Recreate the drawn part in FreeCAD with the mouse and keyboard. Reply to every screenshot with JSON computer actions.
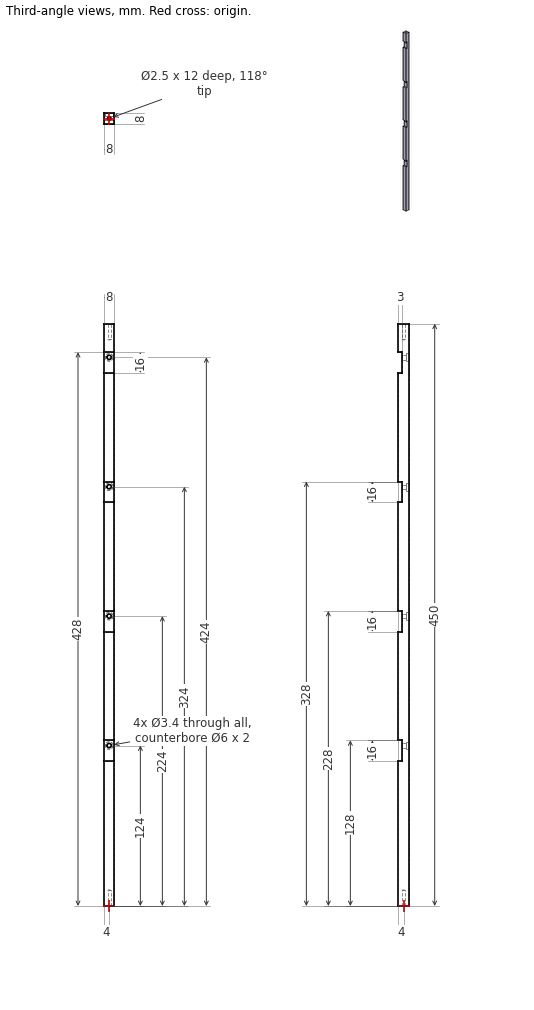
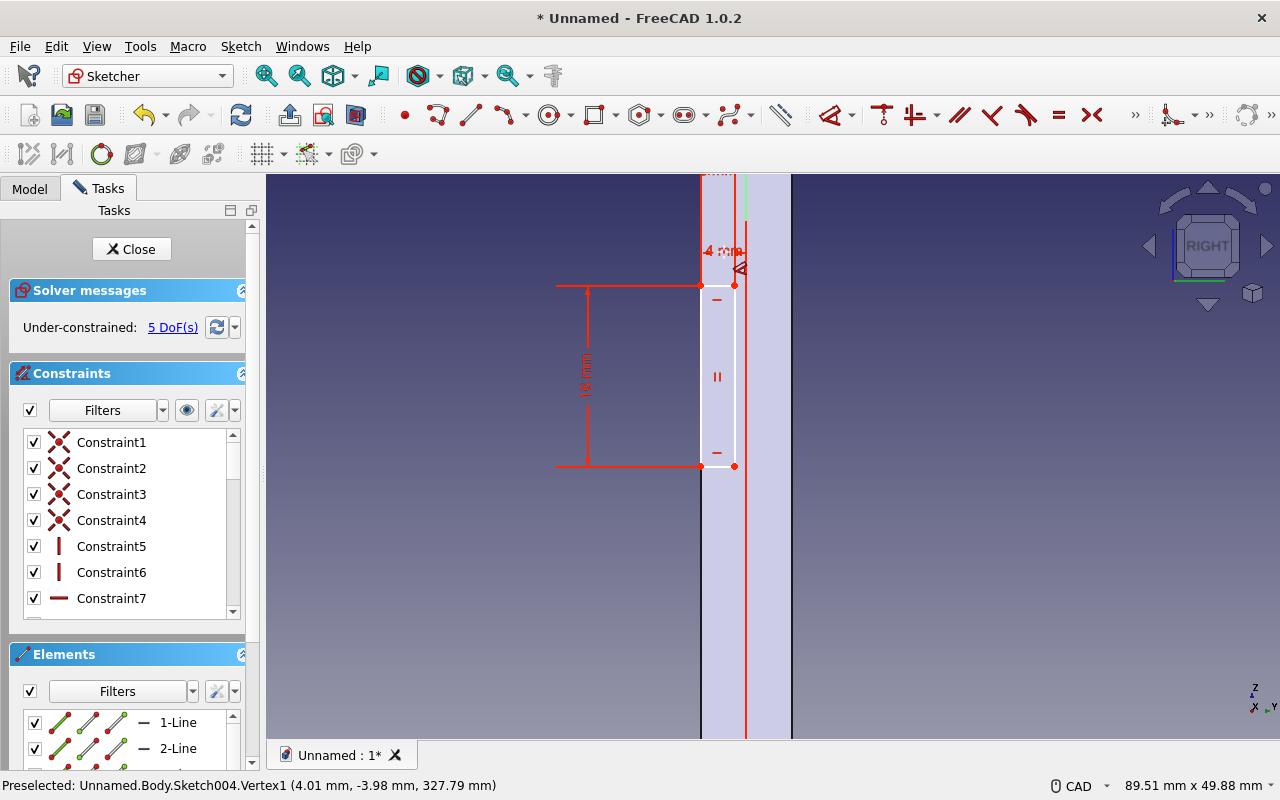
{"action": "scroll", "coordinate": [703, 288], "scroll_direction": "down", "scroll_amount": 12}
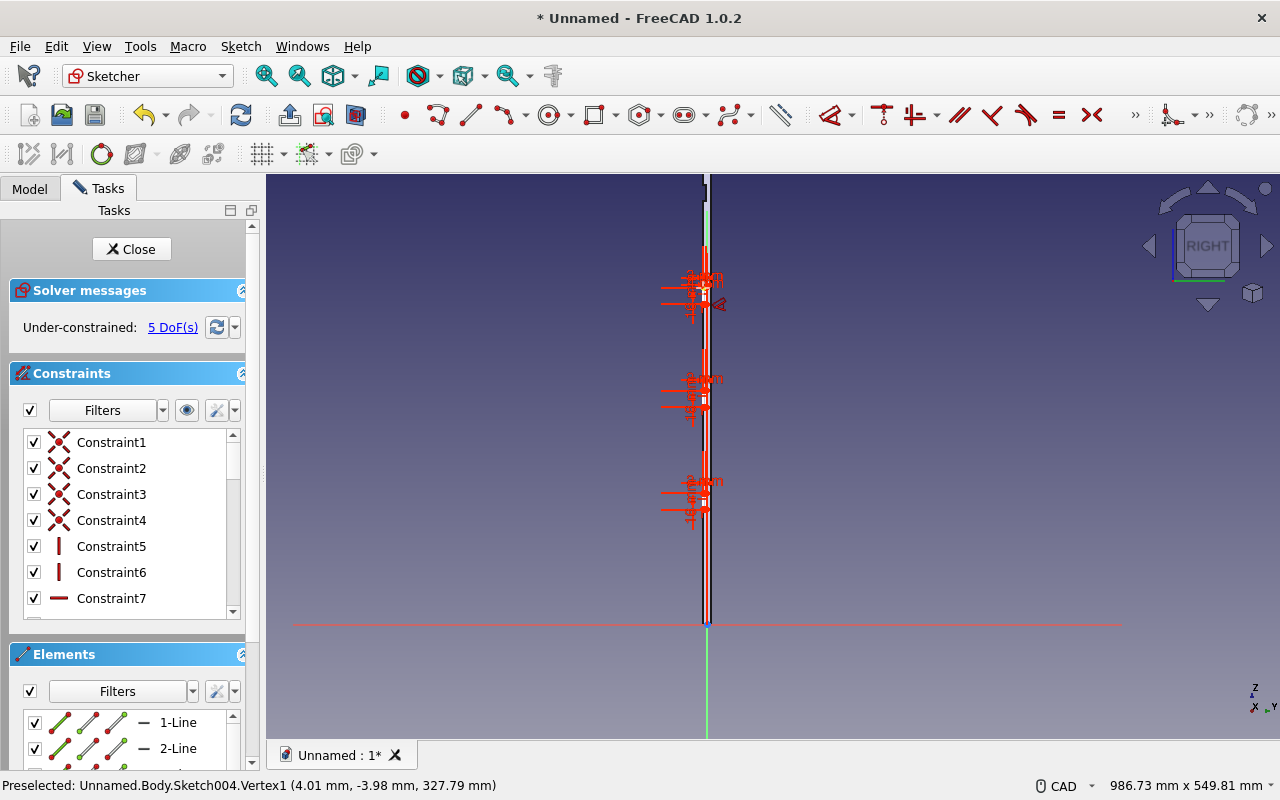
{"action": "scroll", "coordinate": [703, 391], "scroll_direction": "up", "scroll_amount": 12}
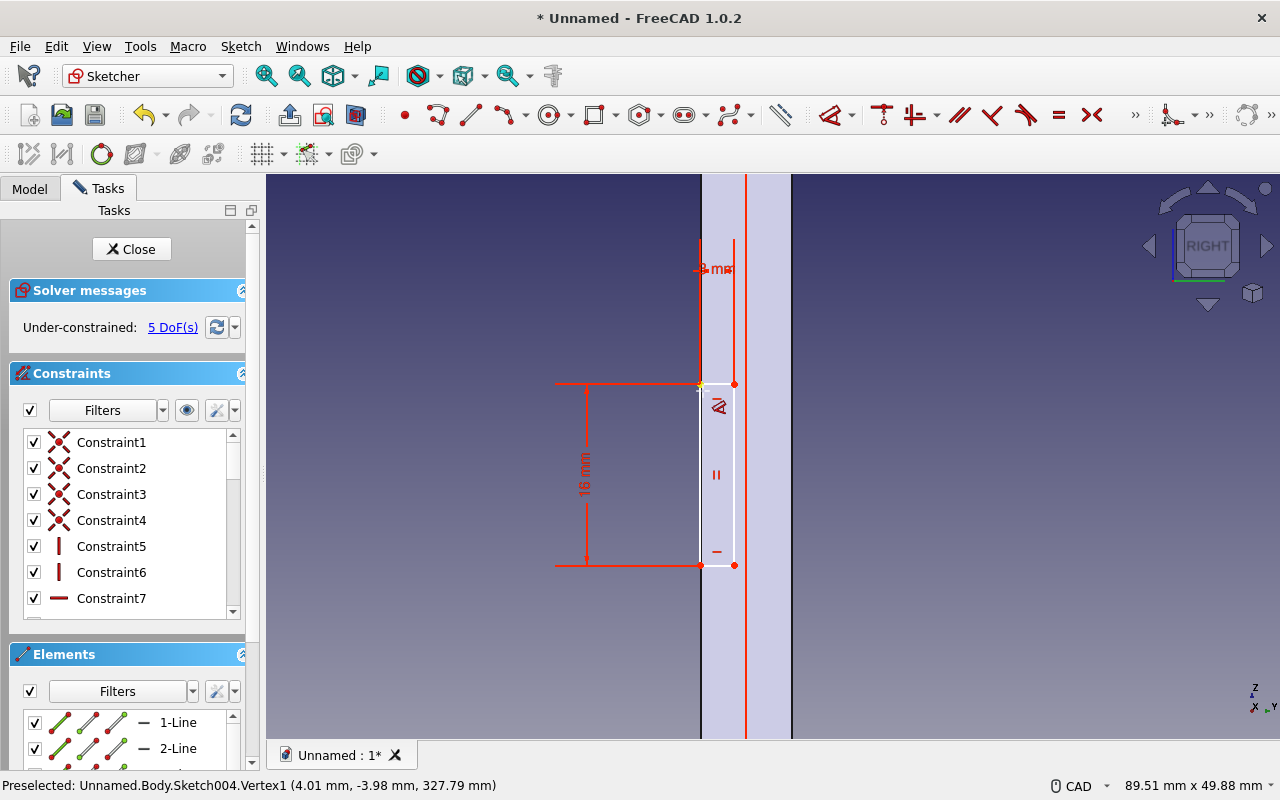
{"action": "left_click", "coordinate": [700, 384]}
{"action": "left_click", "coordinate": [723, 350]}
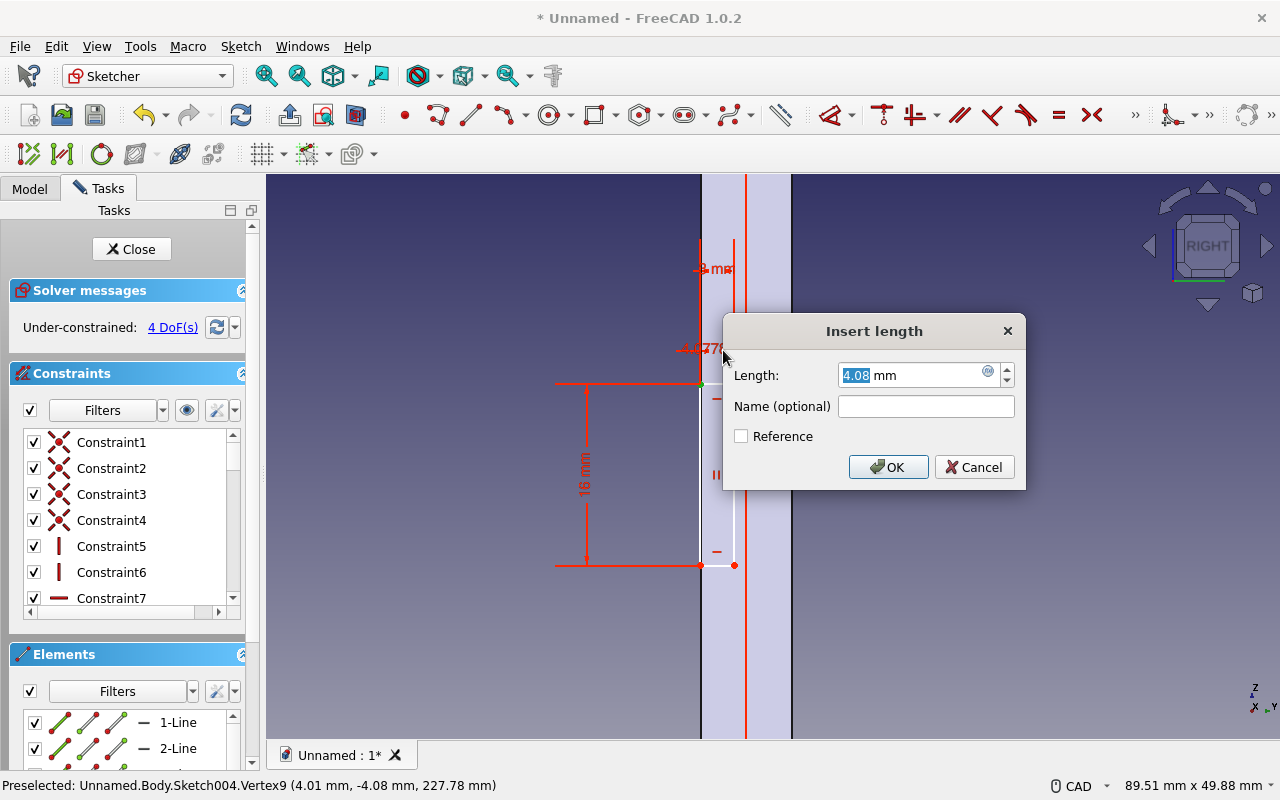
{"action": "type", "text": "4"}
{"action": "key", "text": "Return"}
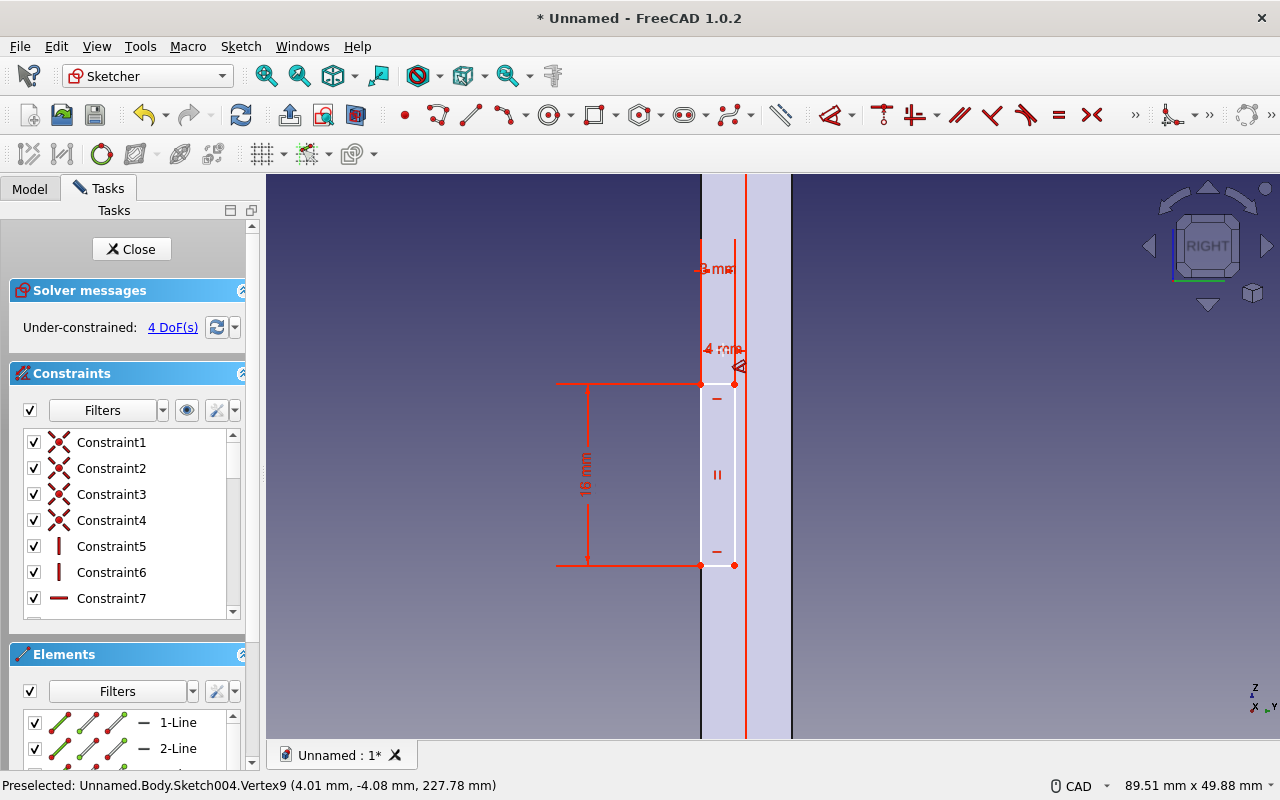
{"action": "scroll", "coordinate": [703, 392], "scroll_direction": "down", "scroll_amount": 12}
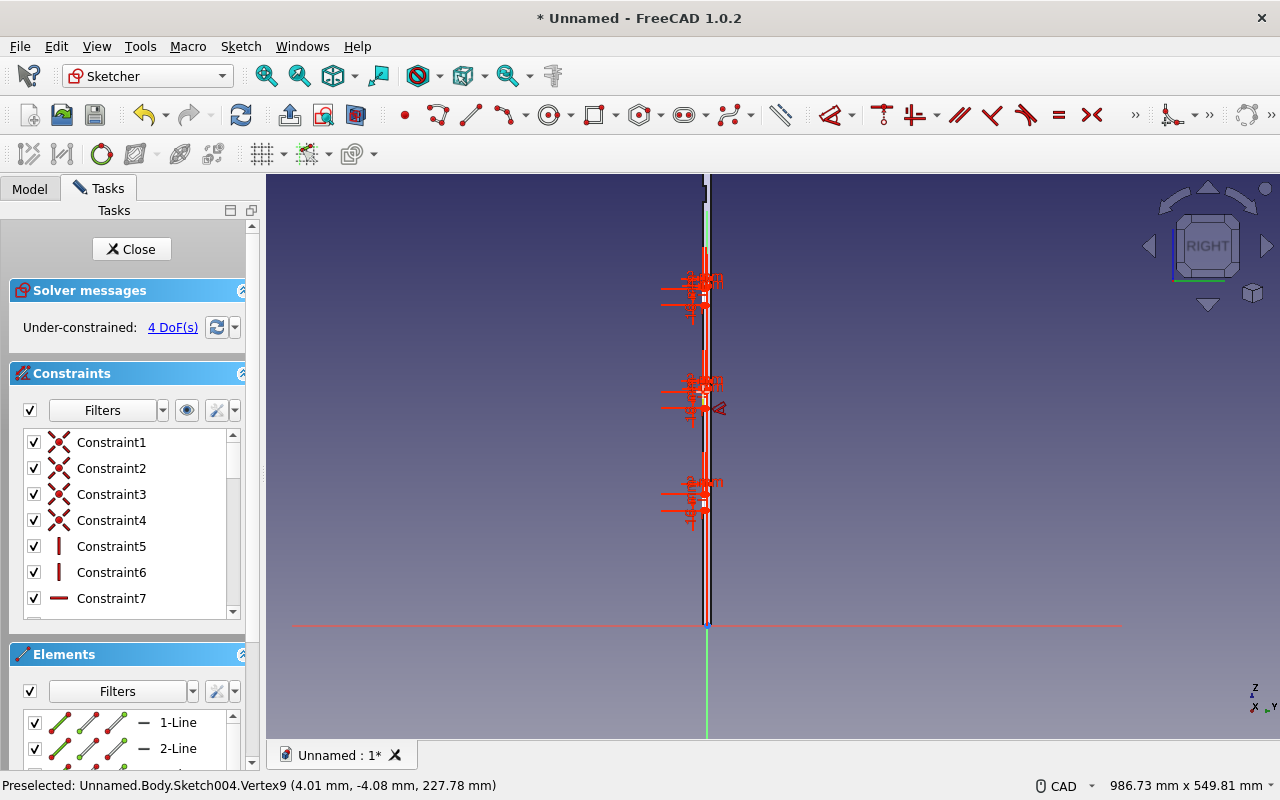
{"action": "scroll", "coordinate": [703, 494], "scroll_direction": "up", "scroll_amount": 12}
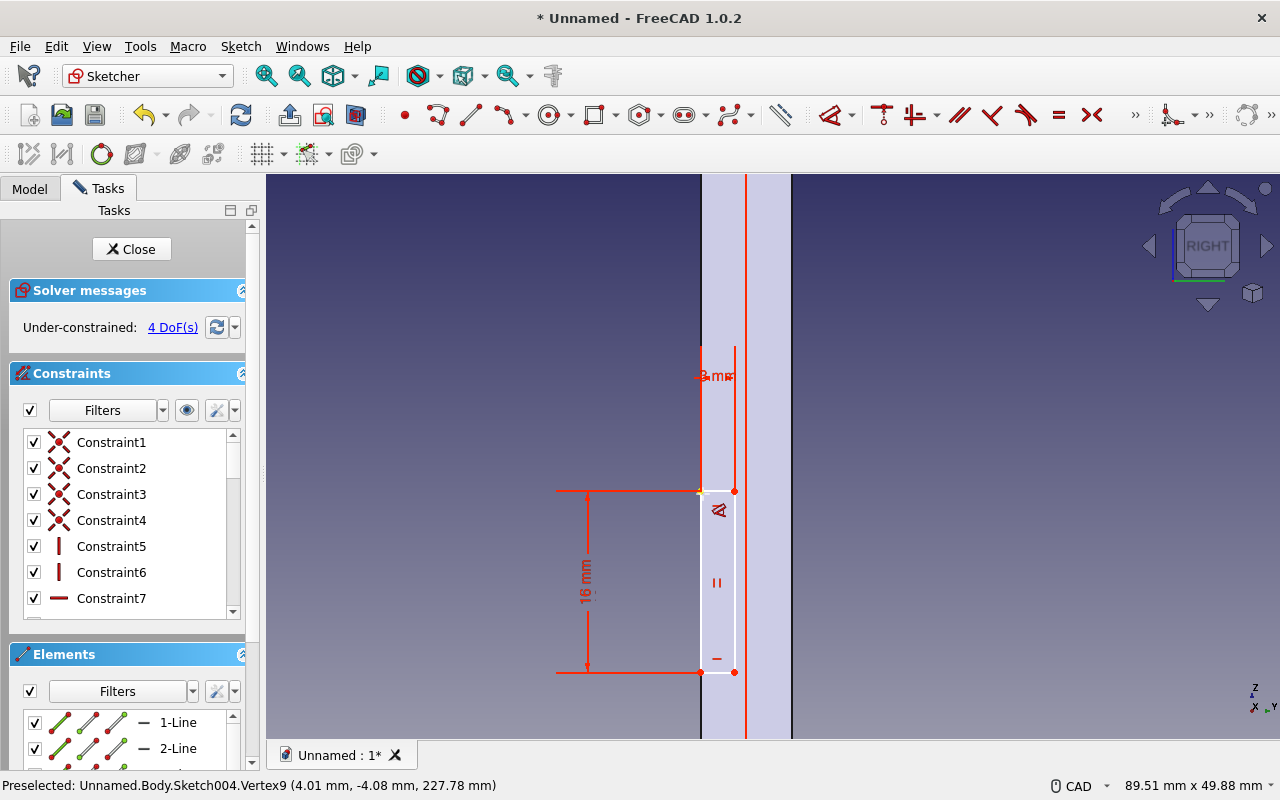
{"action": "left_click", "coordinate": [701, 491]}
{"action": "left_click", "coordinate": [724, 457]}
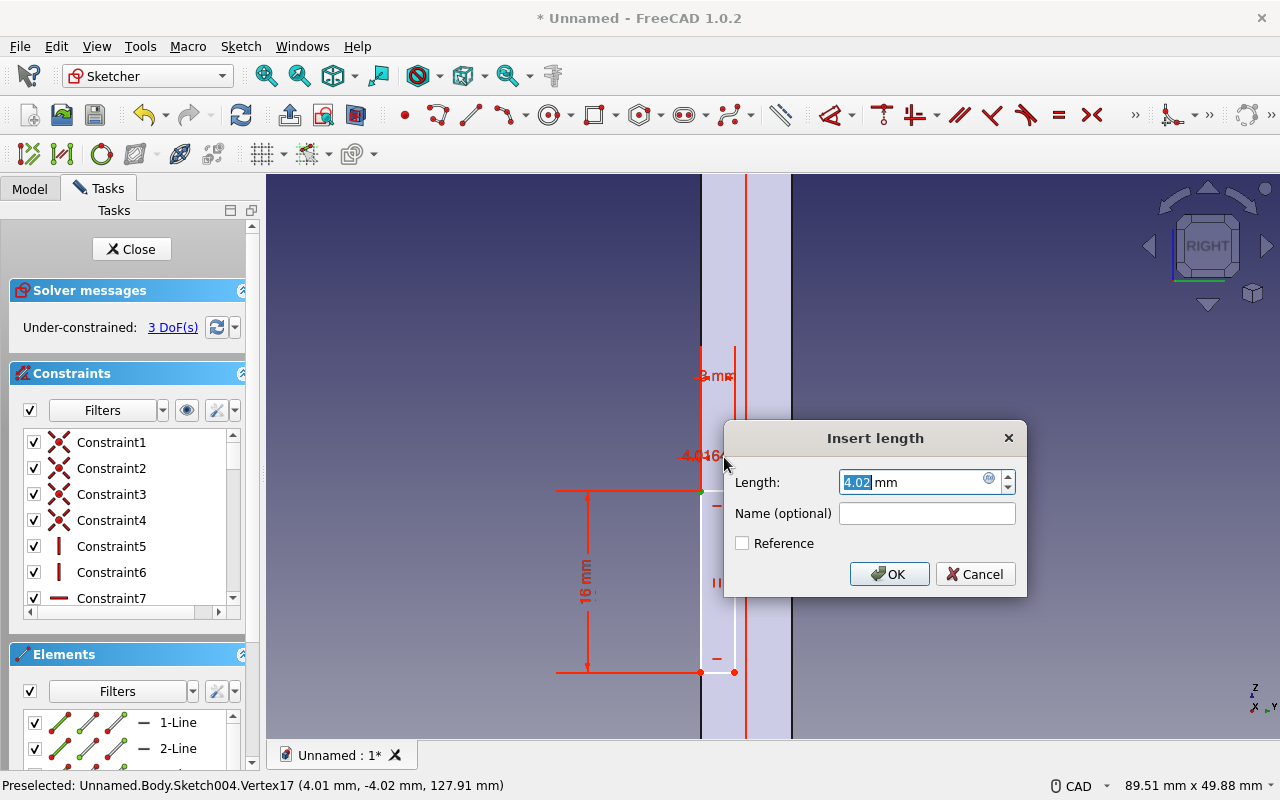
{"action": "type", "text": "4"}
{"action": "key", "text": "Return"}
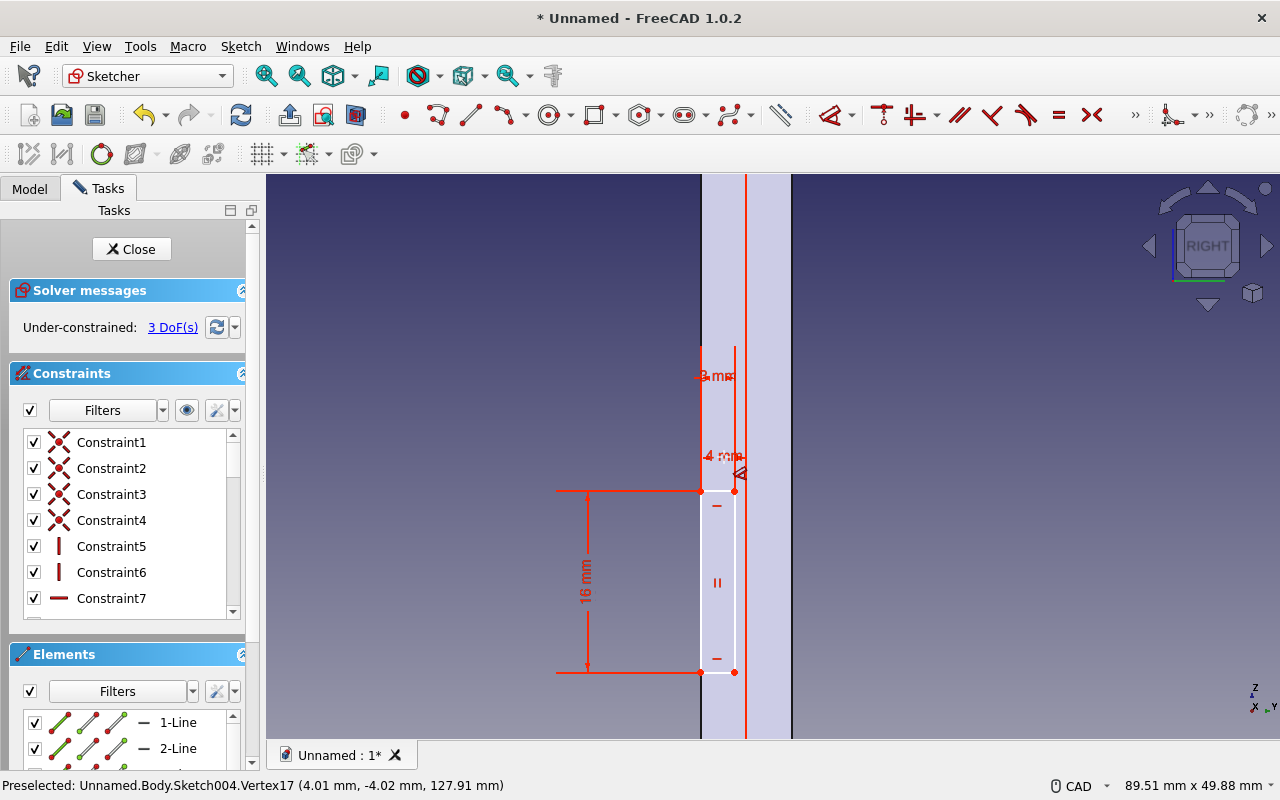
{"action": "scroll", "coordinate": [703, 494], "scroll_direction": "down", "scroll_amount": 12}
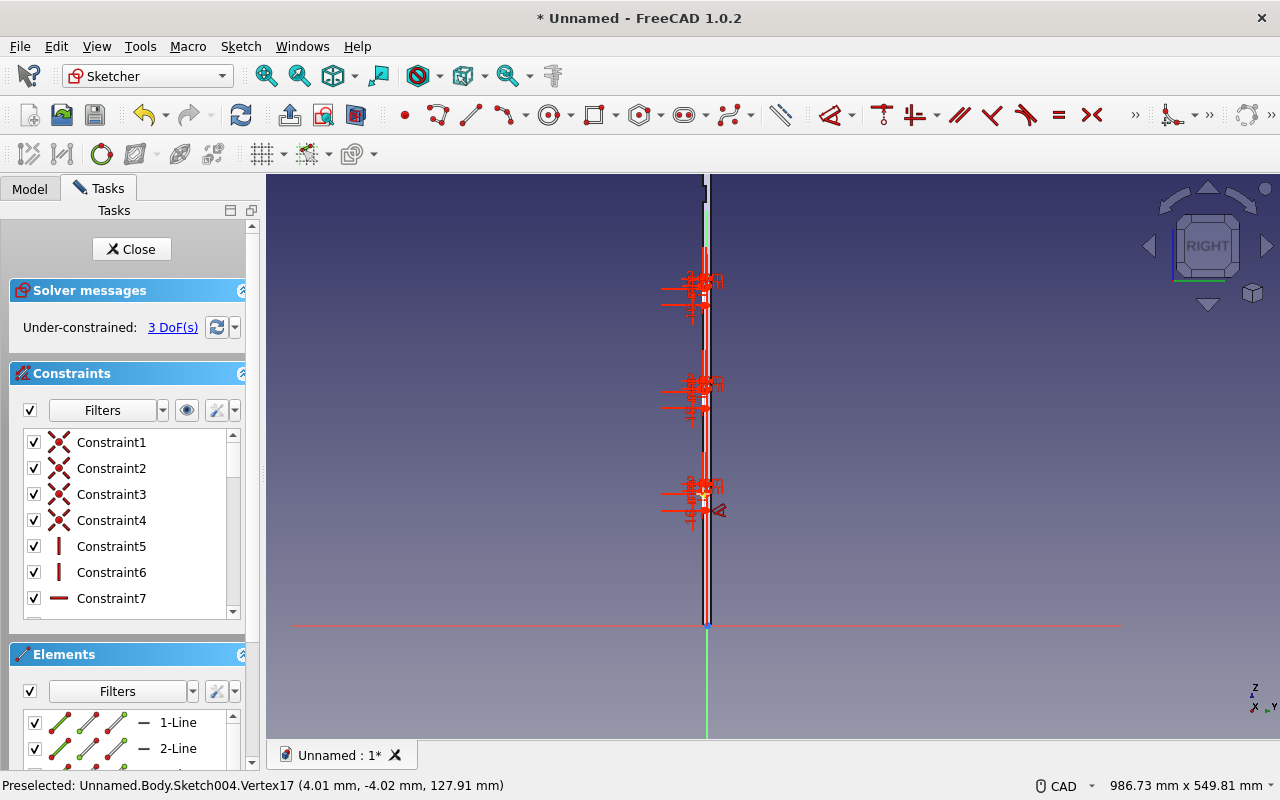
{"action": "scroll", "coordinate": [703, 289], "scroll_direction": "up", "scroll_amount": 7}